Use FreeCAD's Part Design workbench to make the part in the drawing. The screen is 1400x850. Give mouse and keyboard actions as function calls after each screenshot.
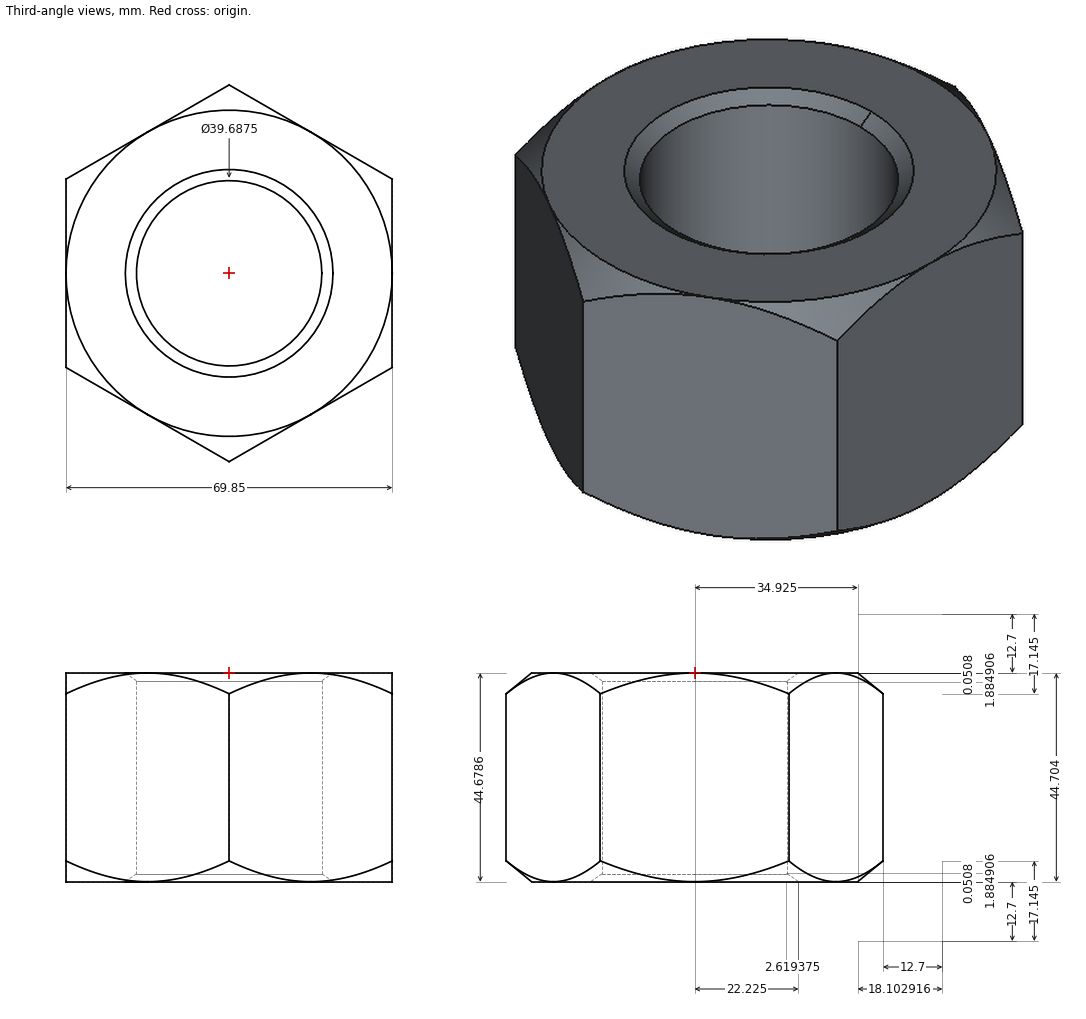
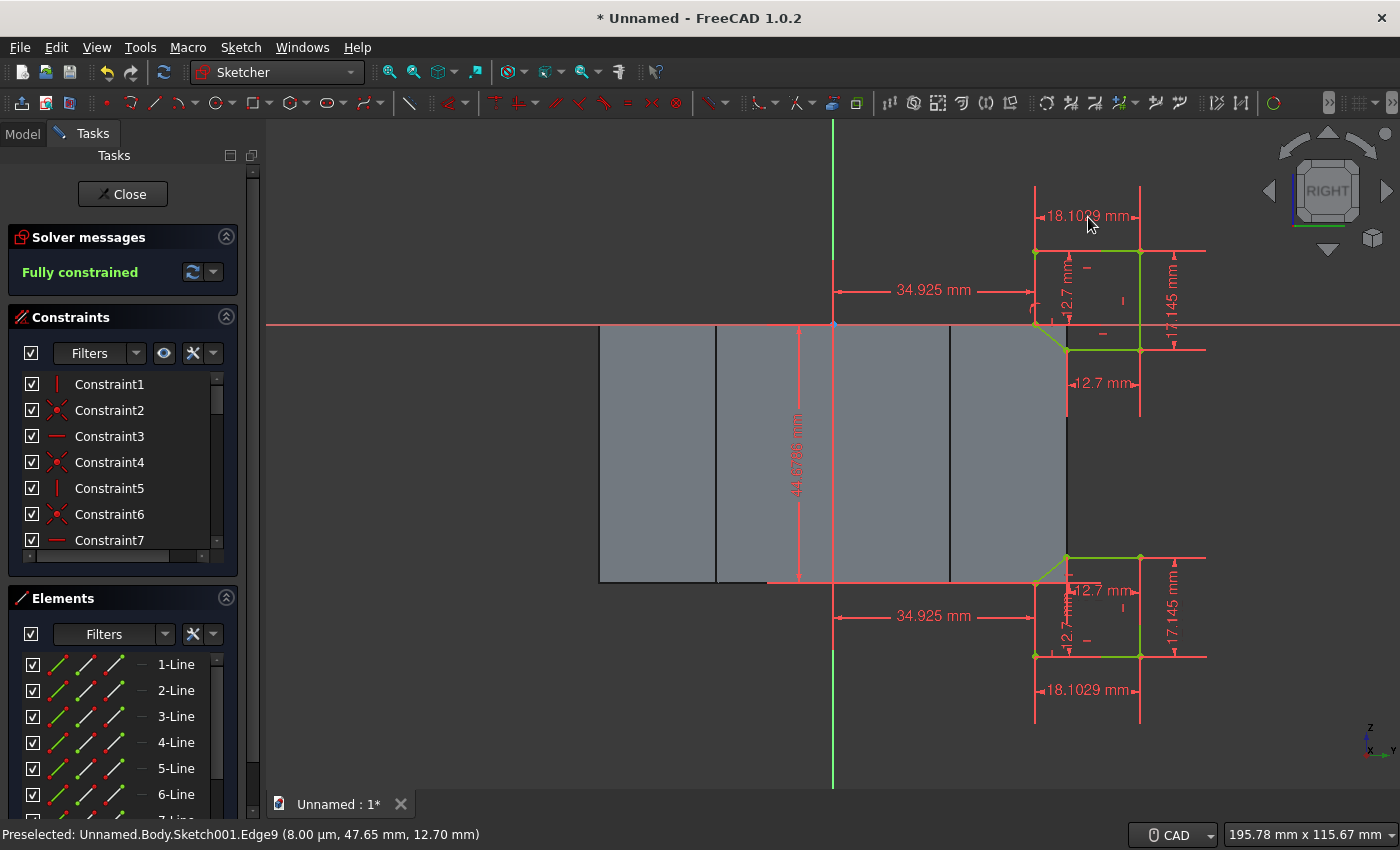
click(123, 194)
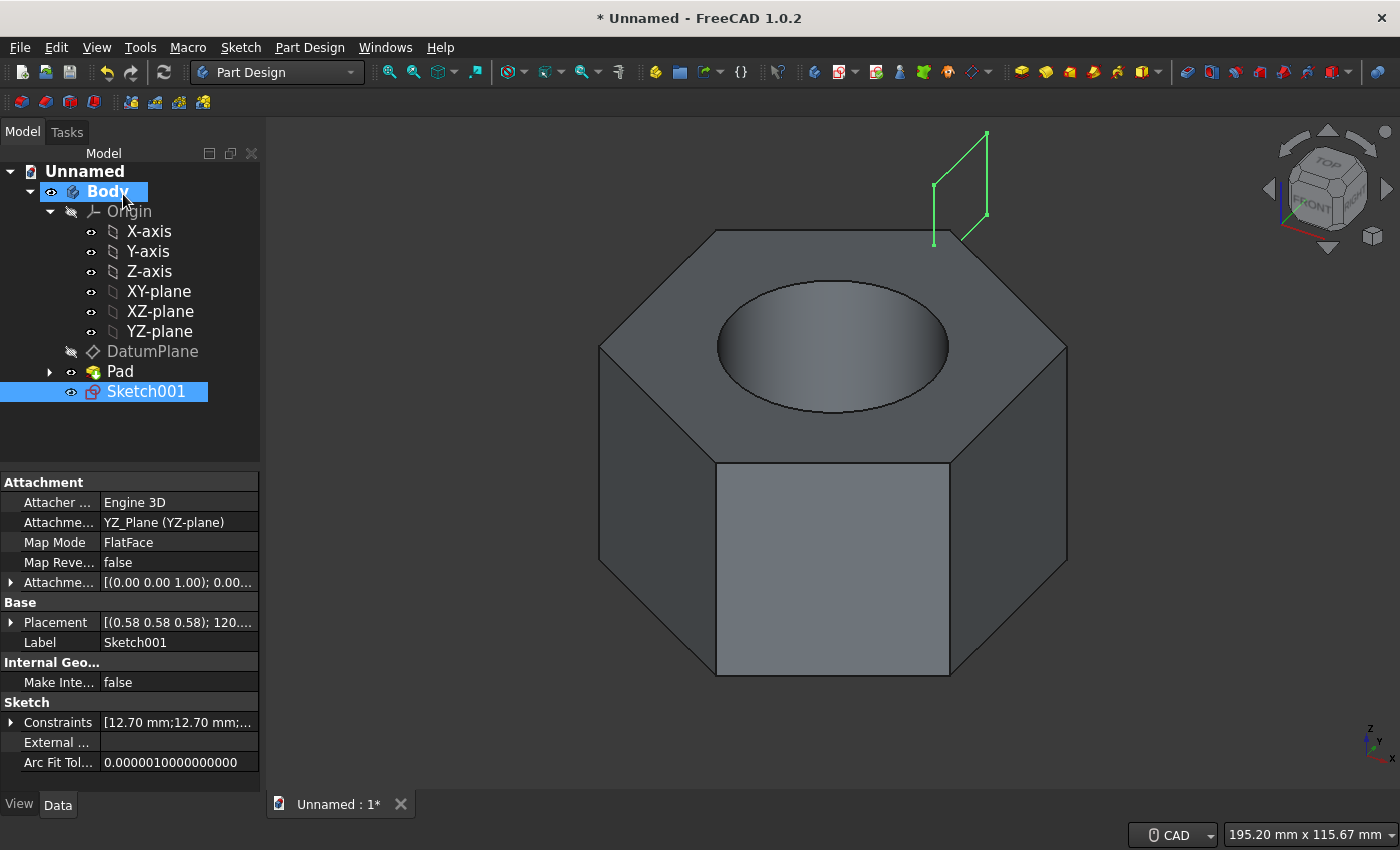
click(1236, 72)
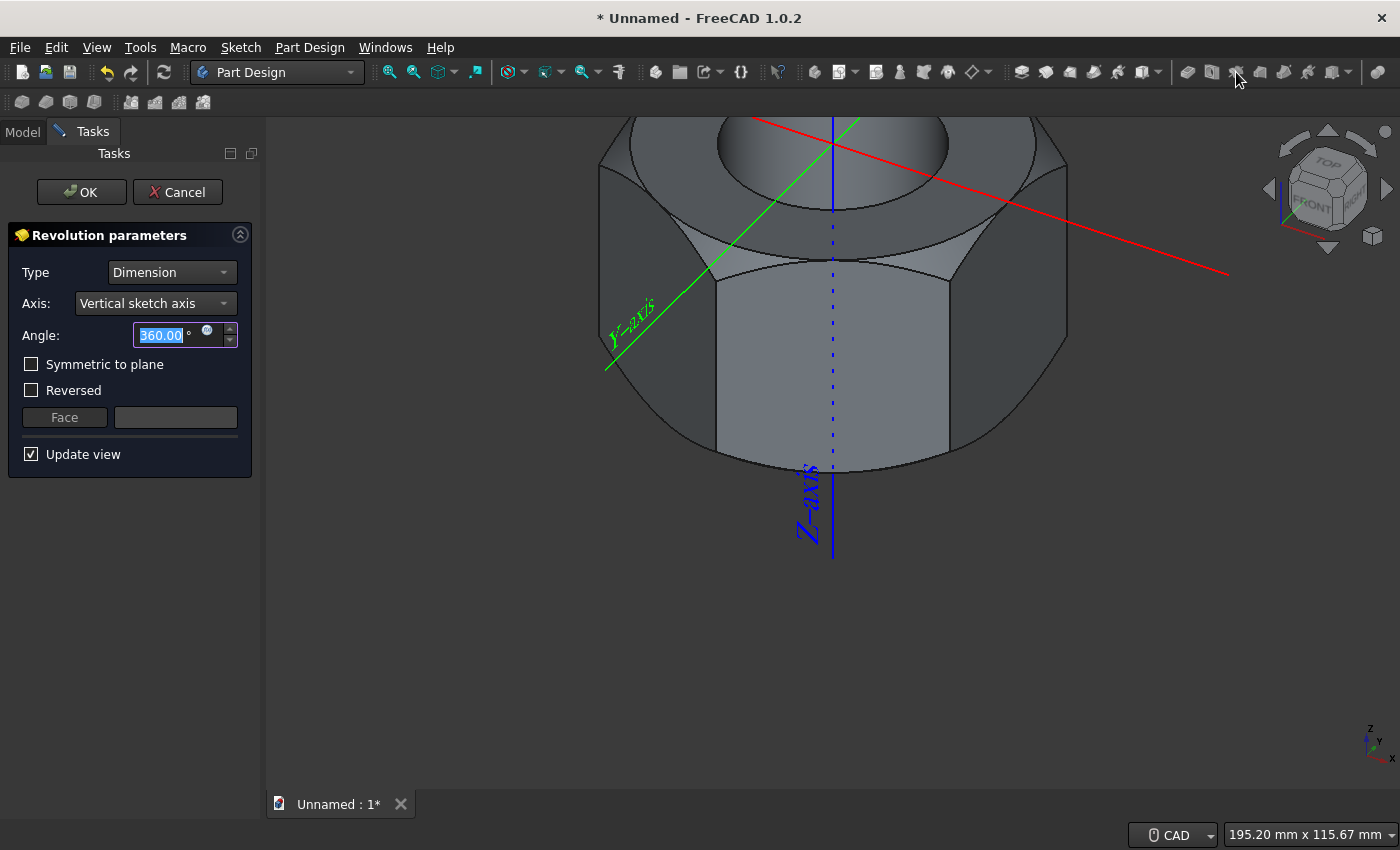
click(82, 192)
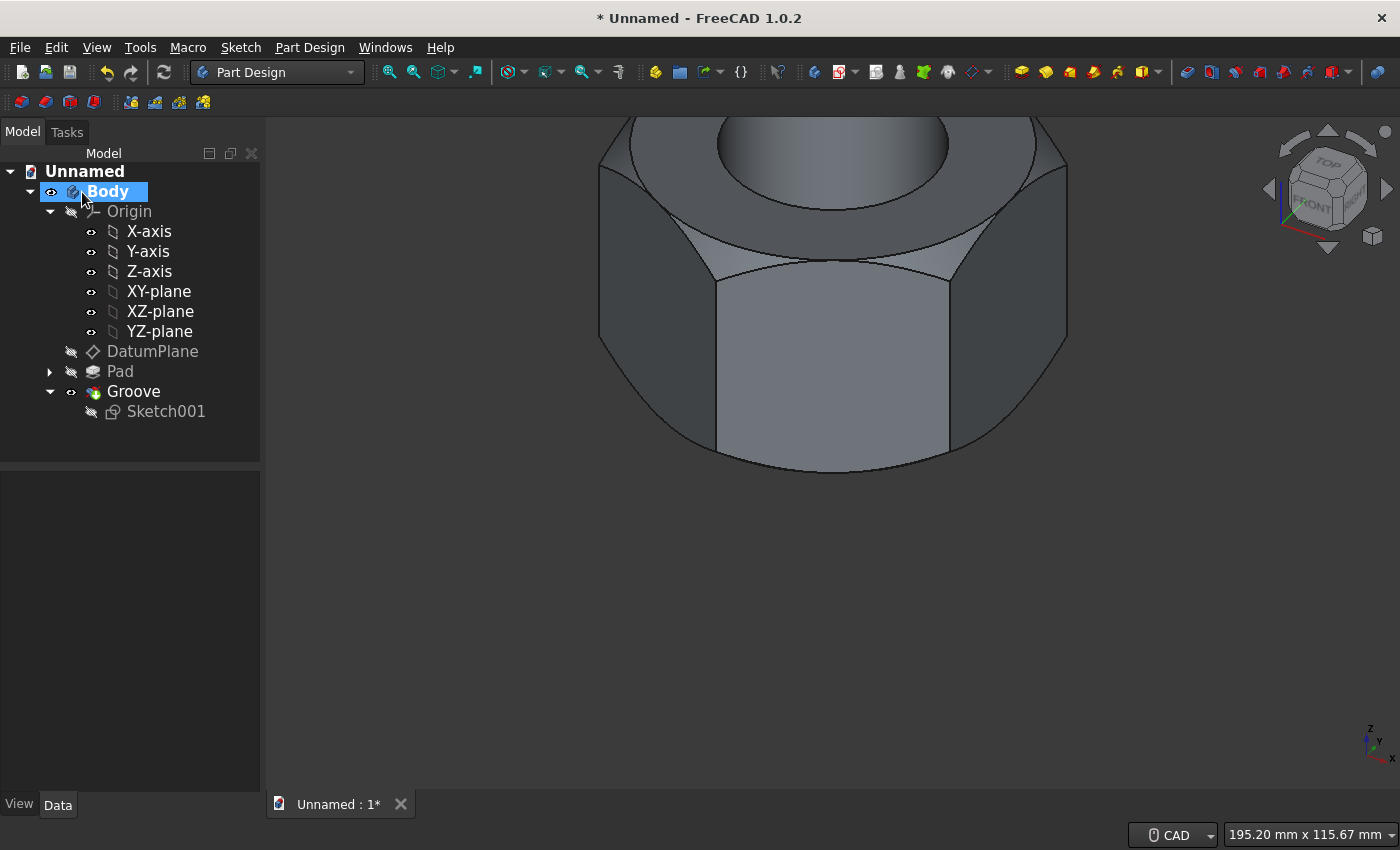
click(390, 72)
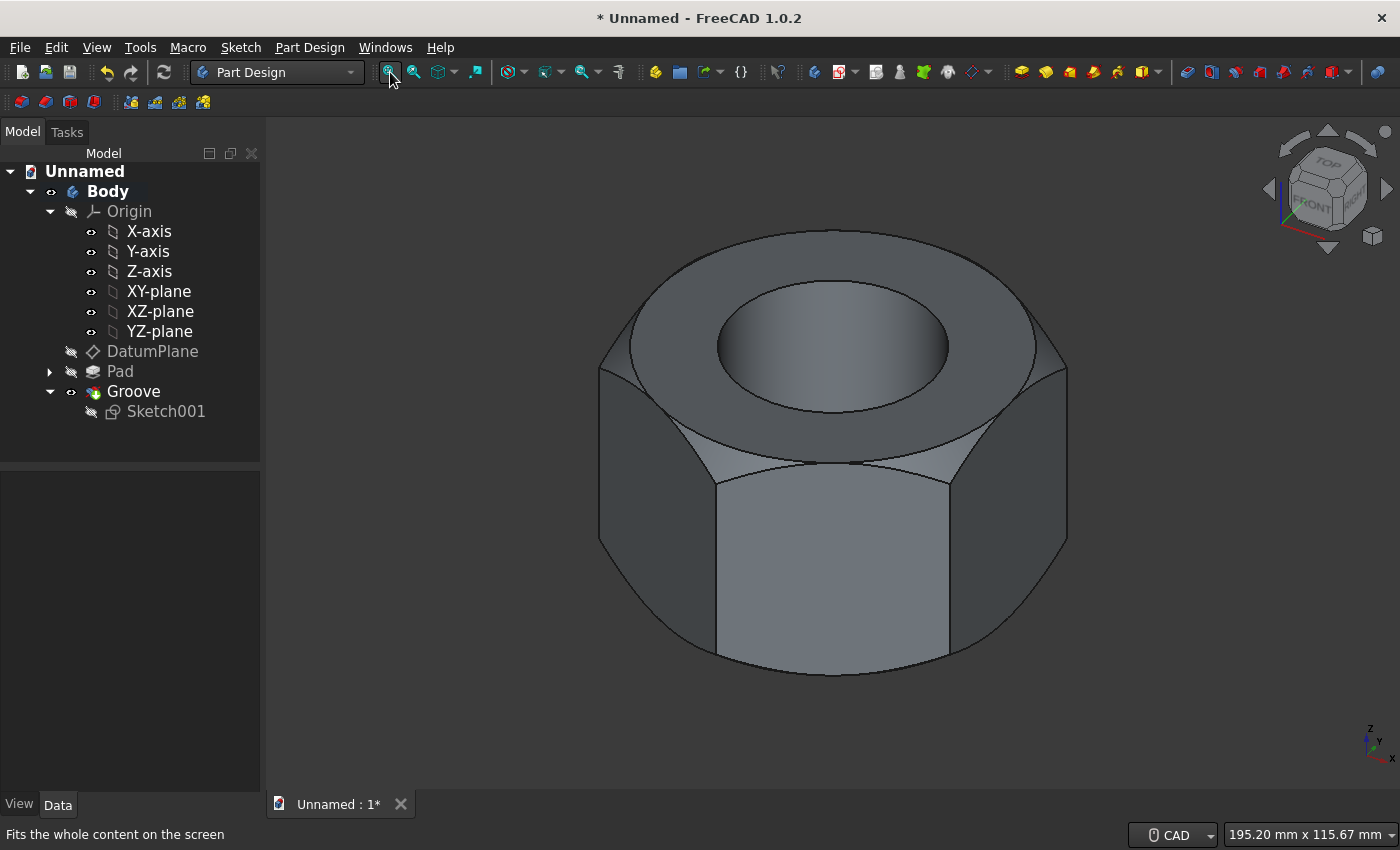
click(840, 72)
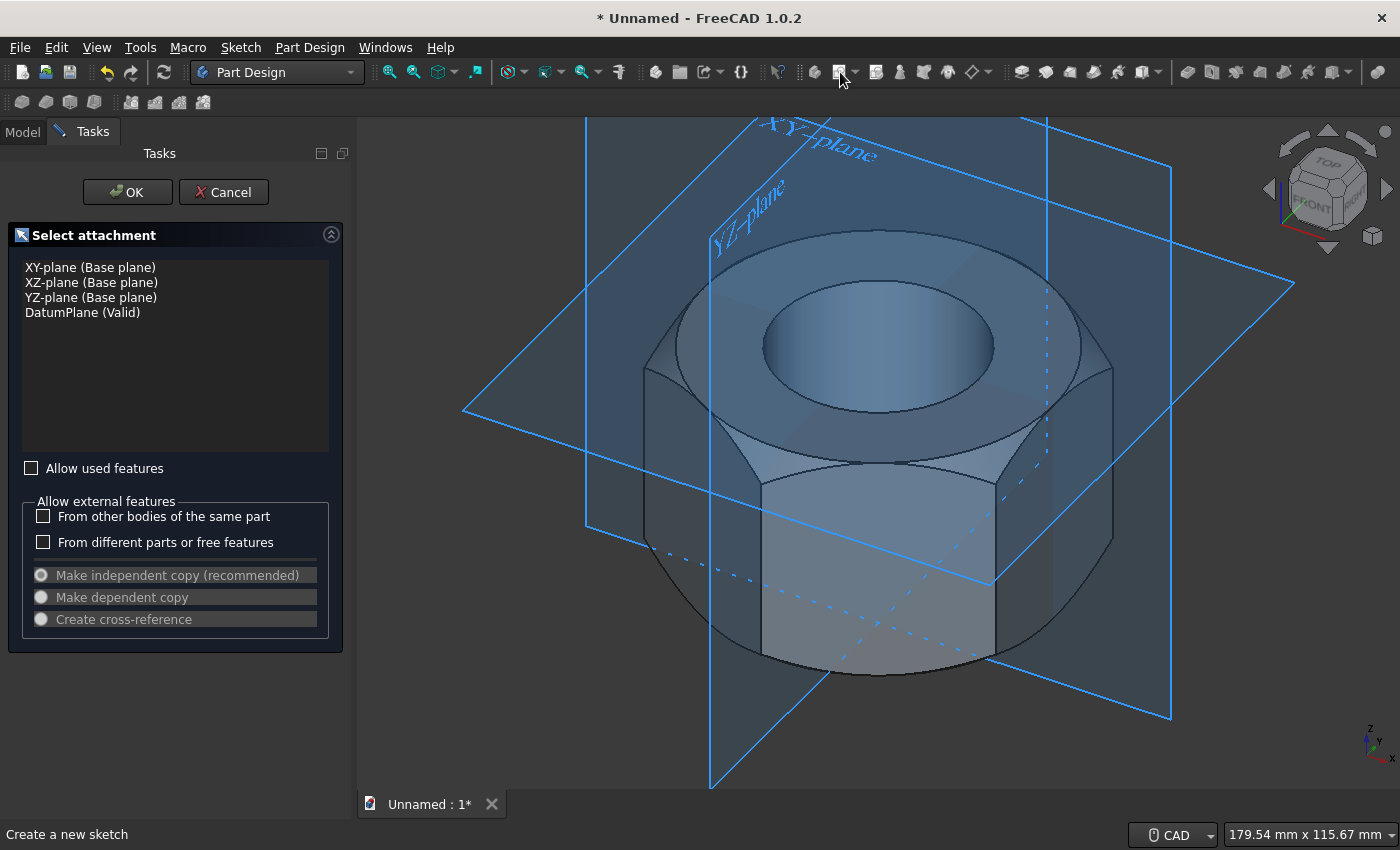
click(82, 298)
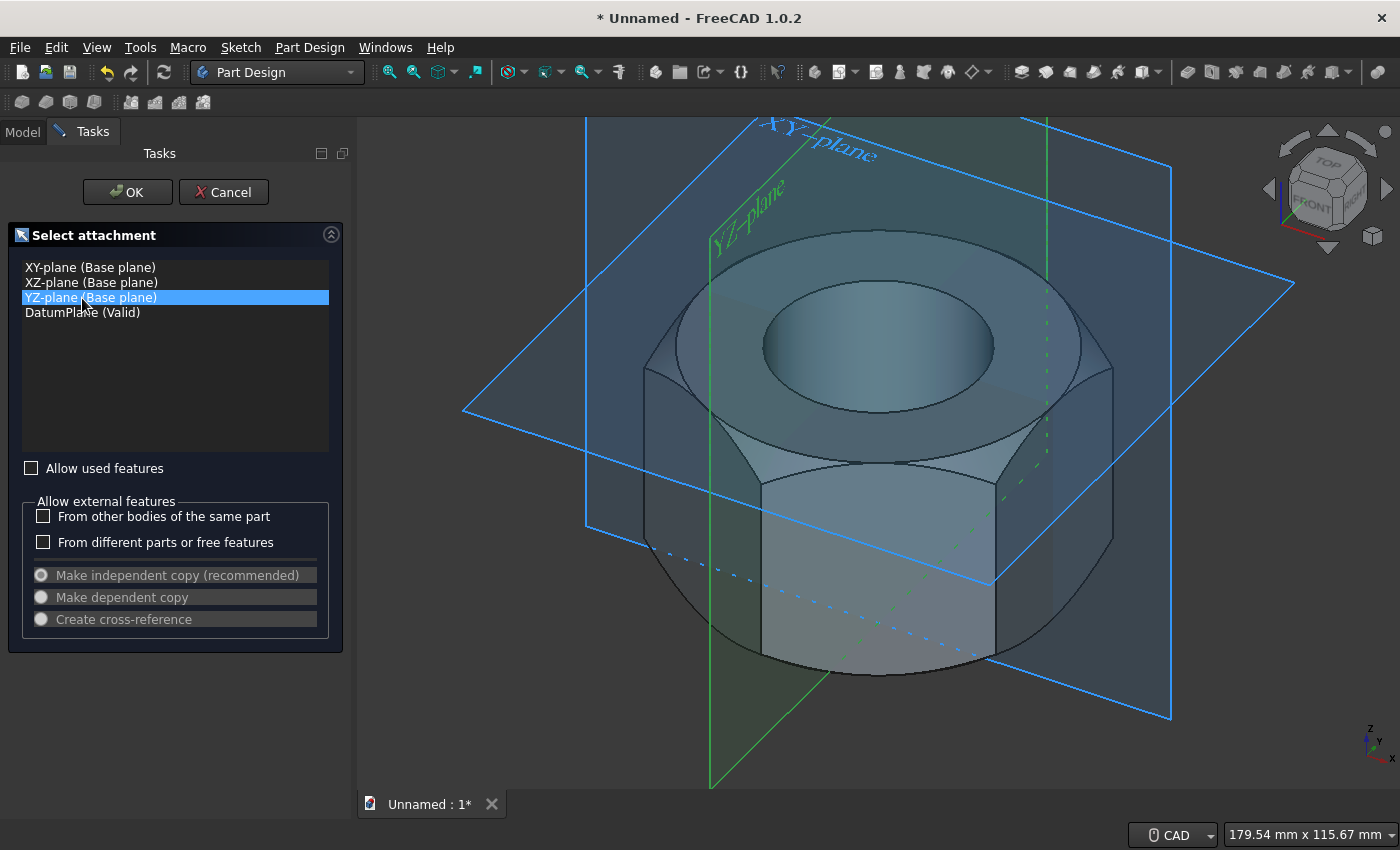
click(128, 192)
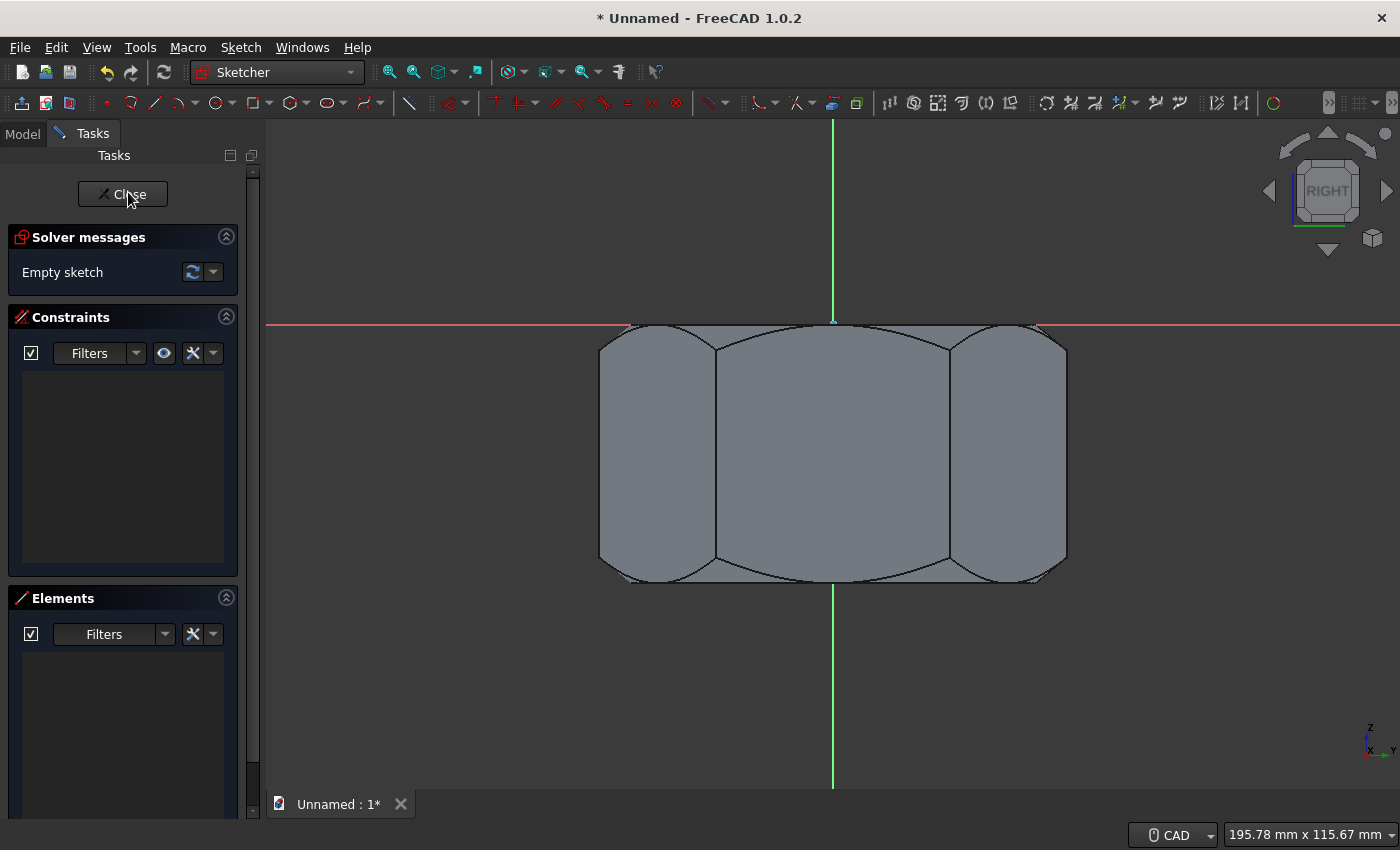
key(q)
key(s)